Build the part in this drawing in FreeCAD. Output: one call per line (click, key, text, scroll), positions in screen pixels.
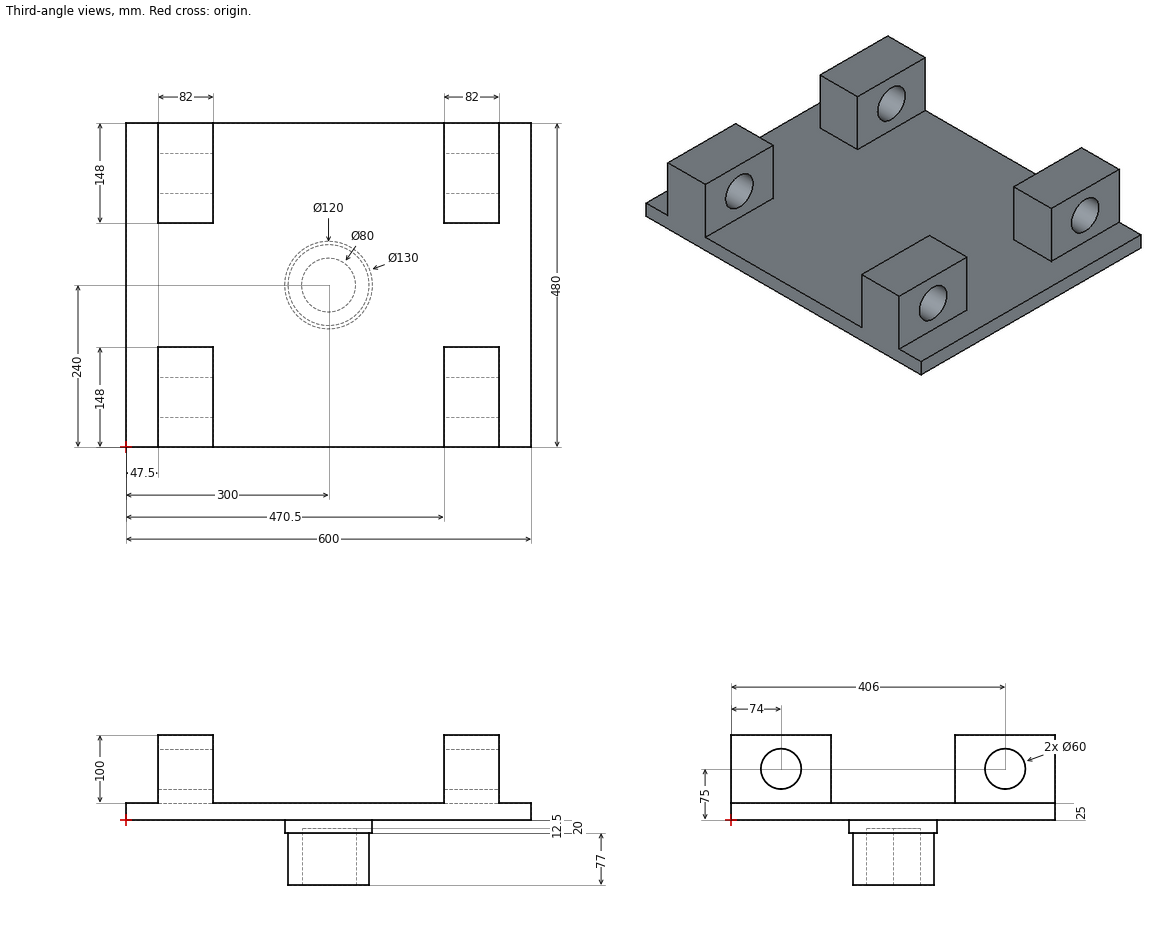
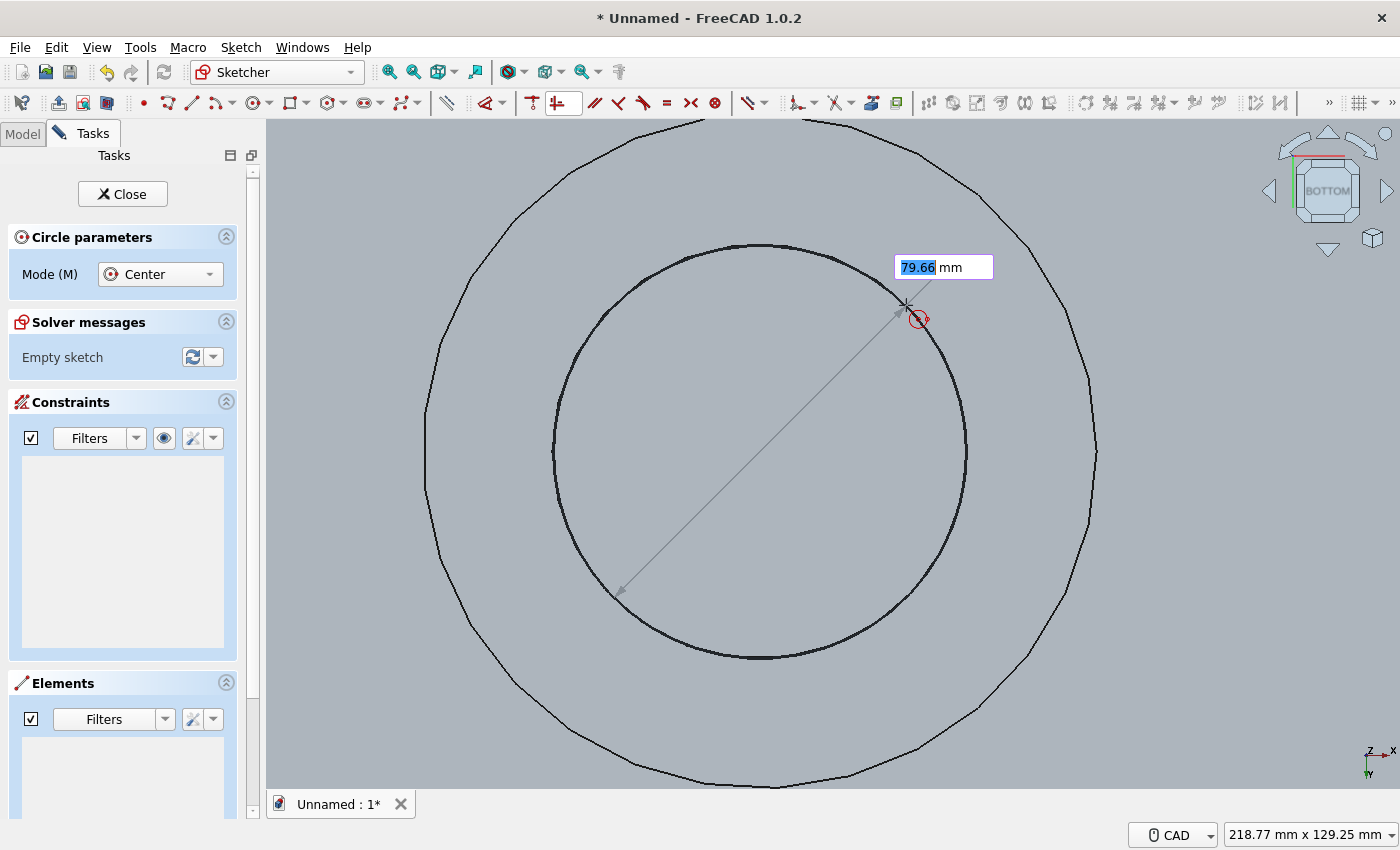
text(80)
key(Return)
key(Escape)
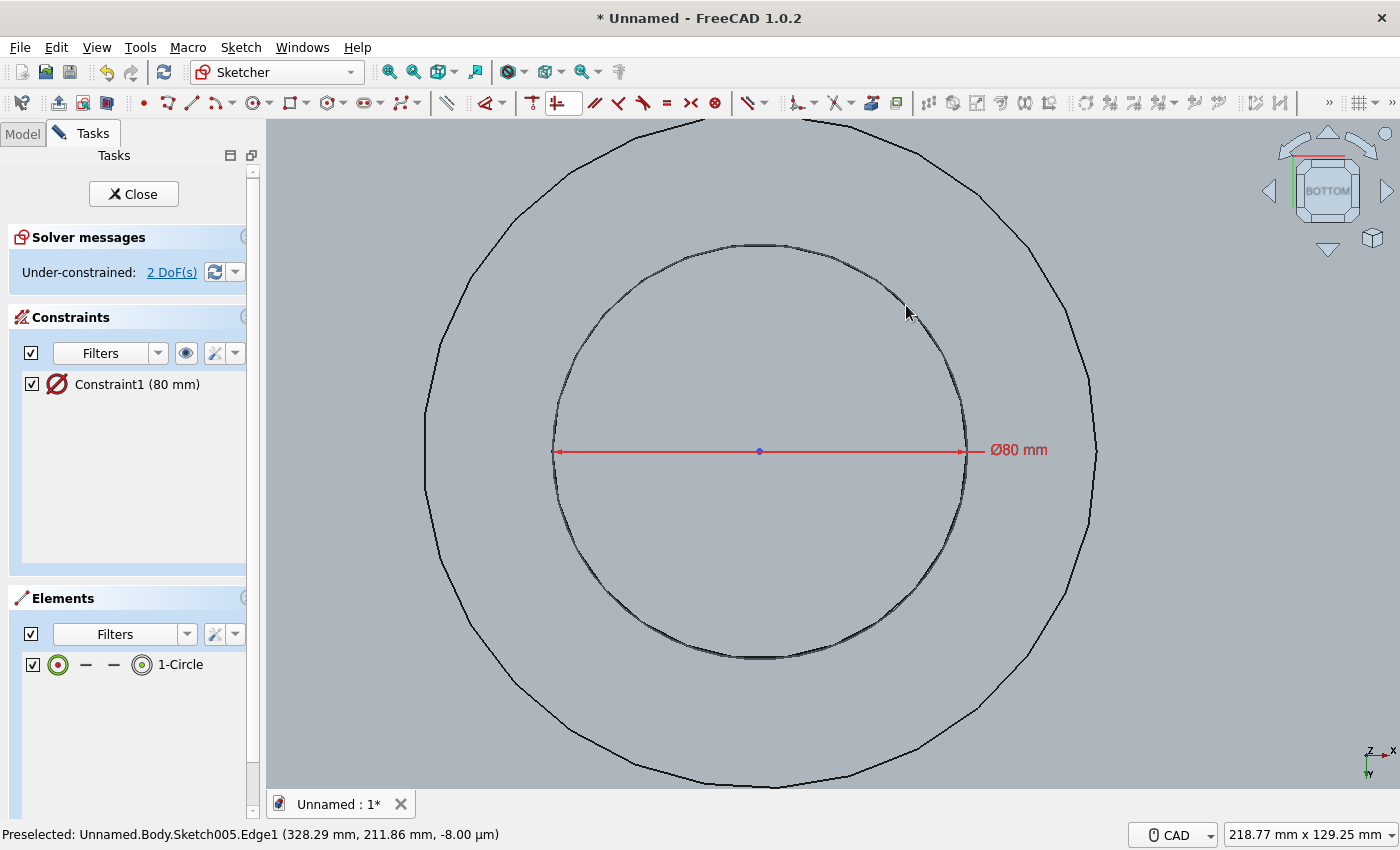
click(486, 104)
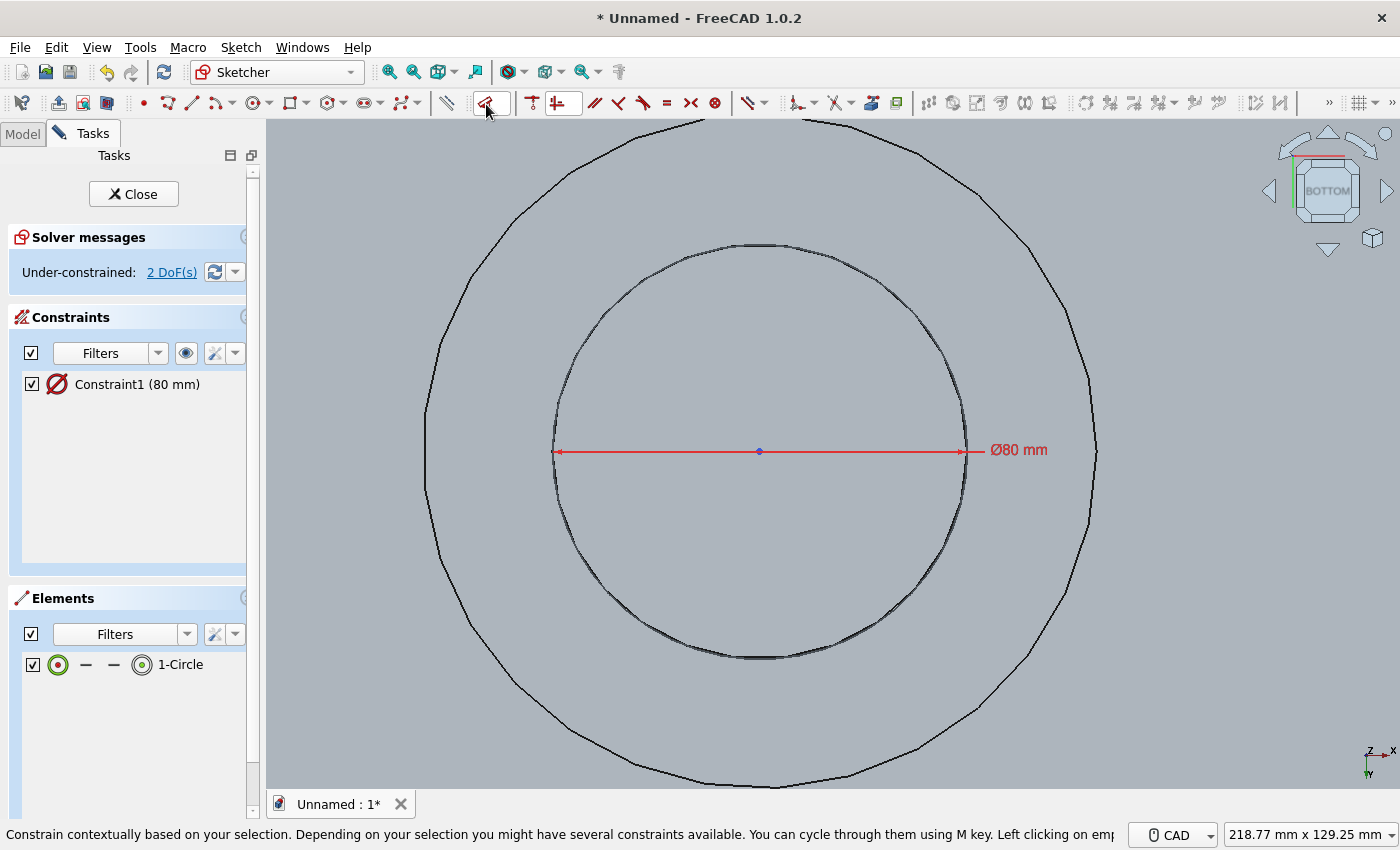
click(760, 452)
click(527, 486)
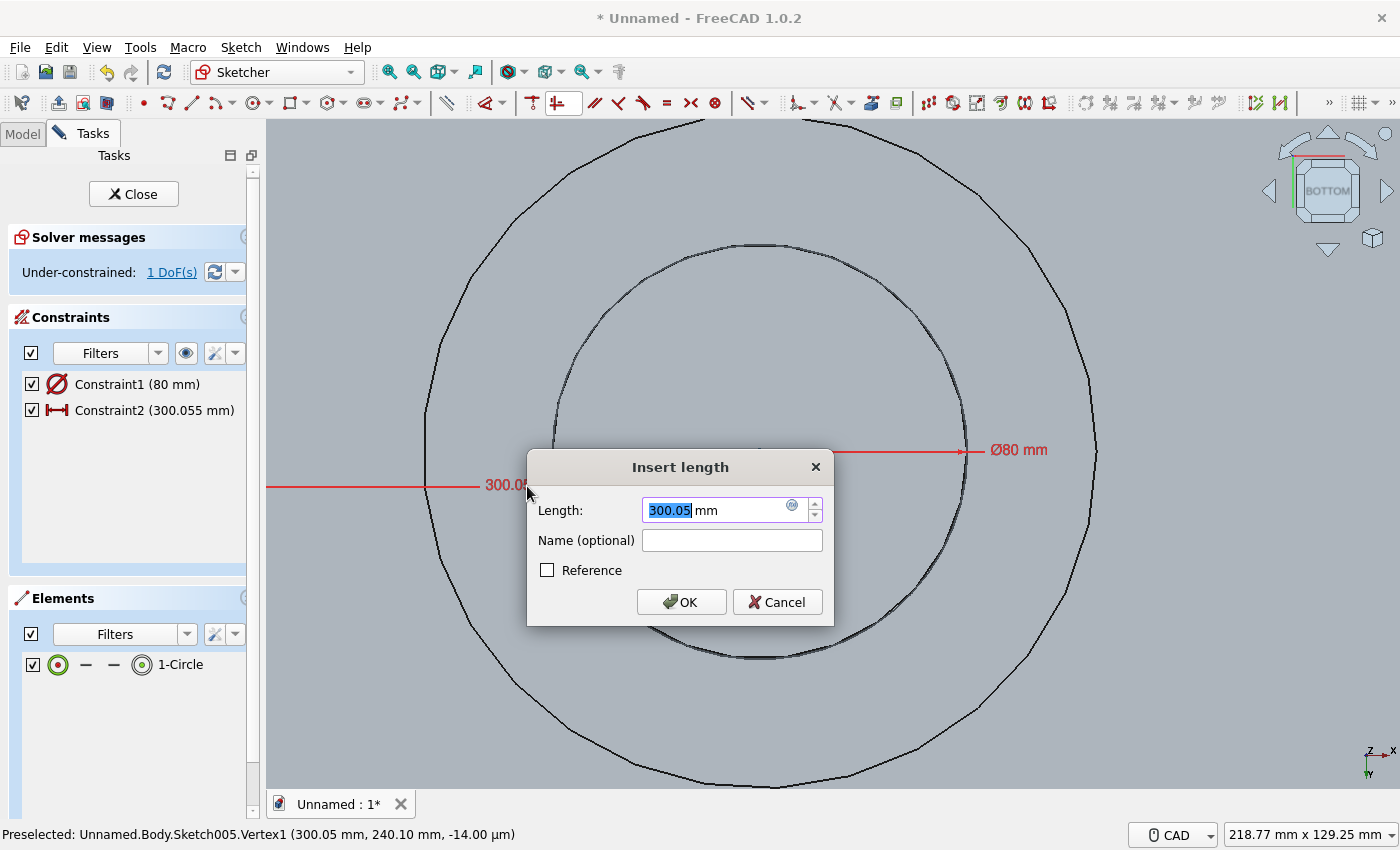
text(300)
key(Return)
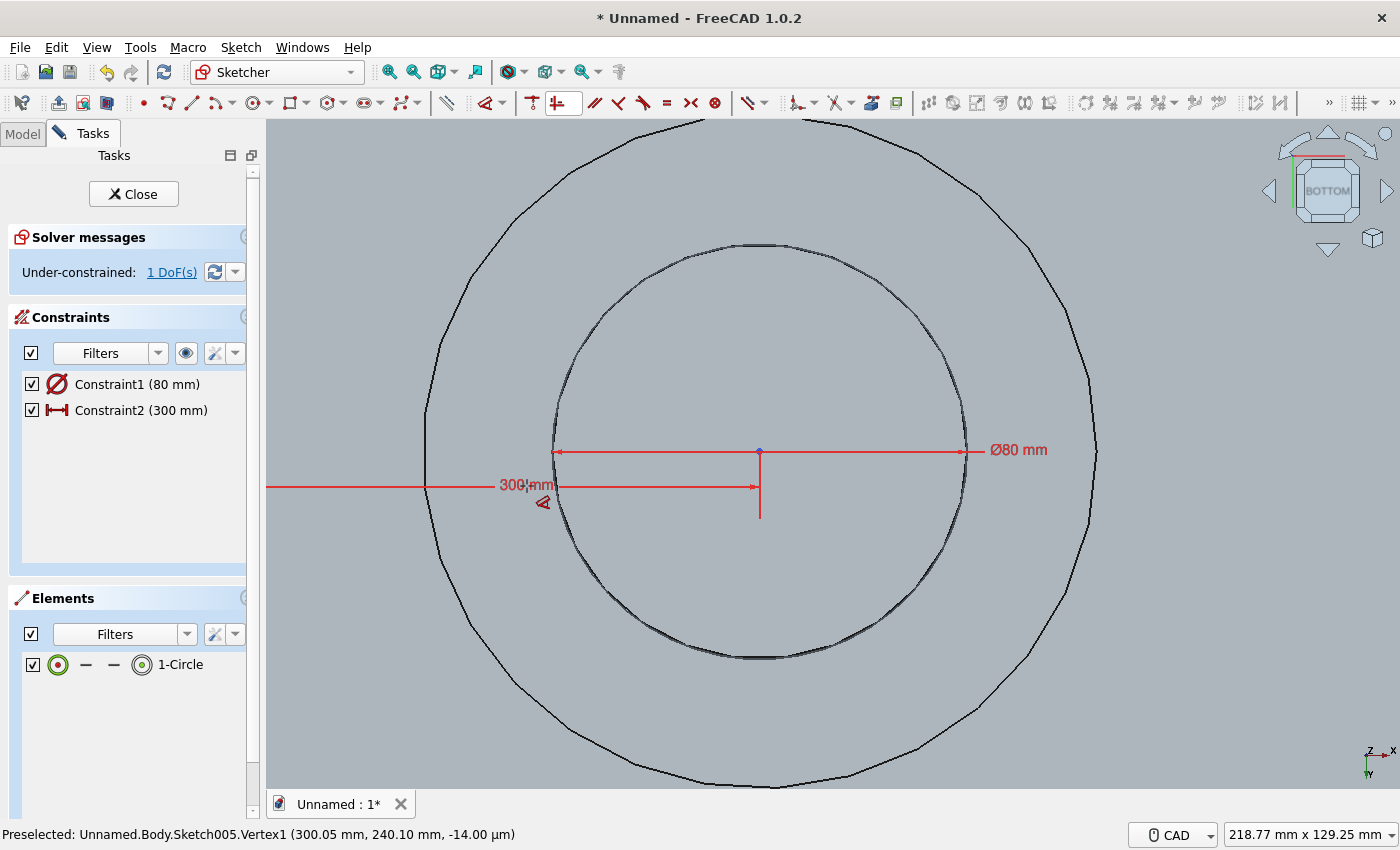
click(760, 452)
click(794, 299)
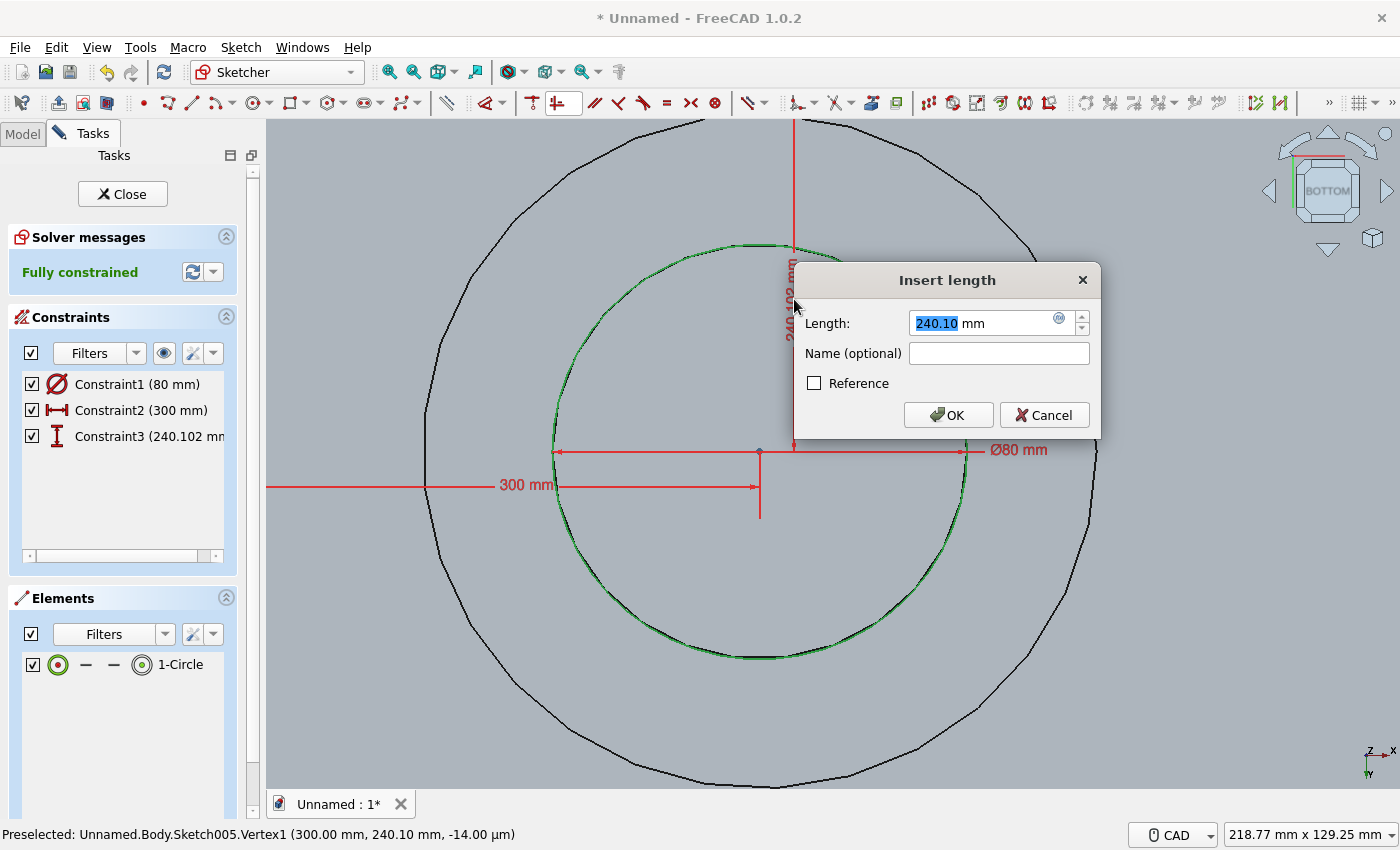
text(240)
key(Return)
key(Escape)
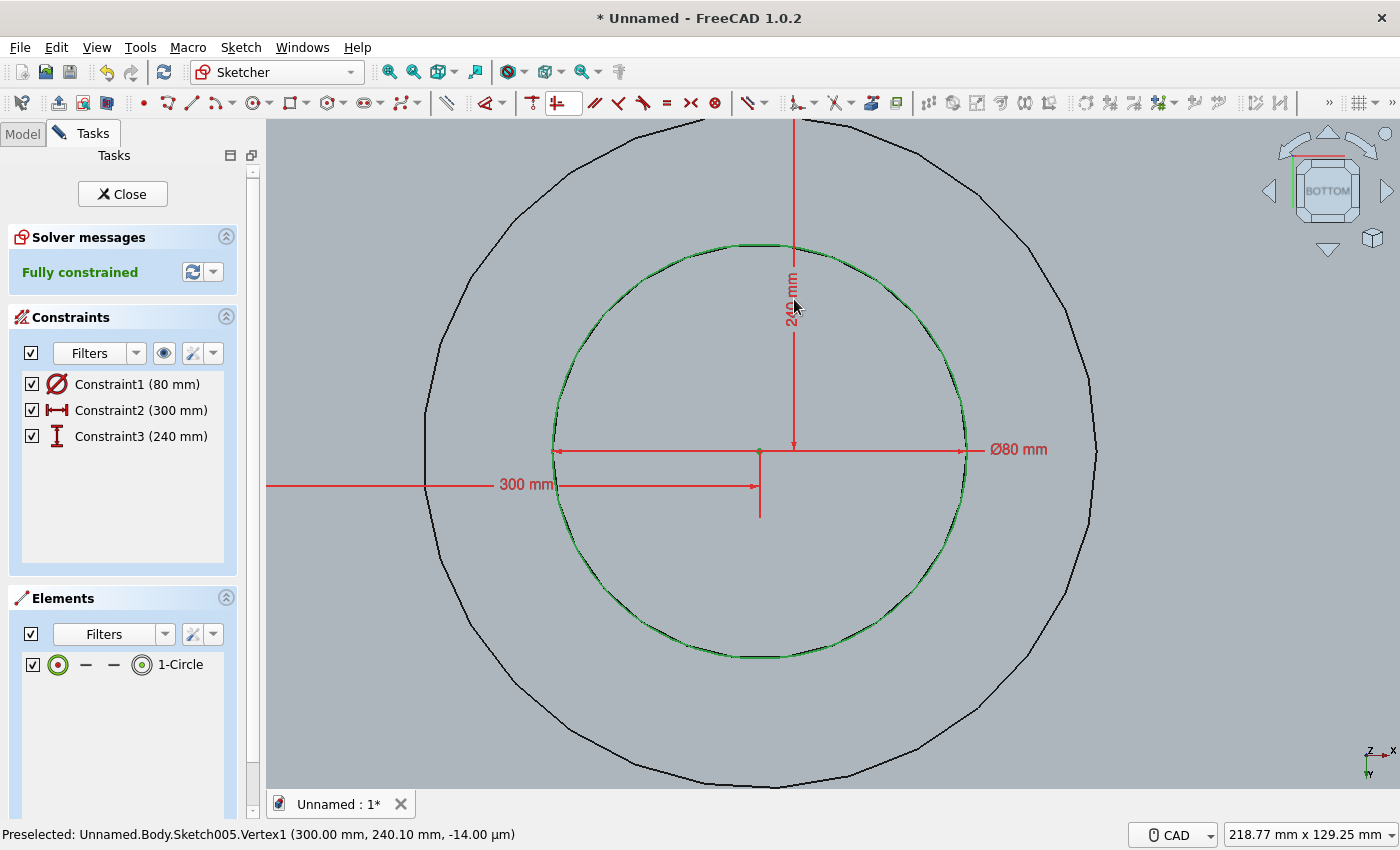
click(123, 194)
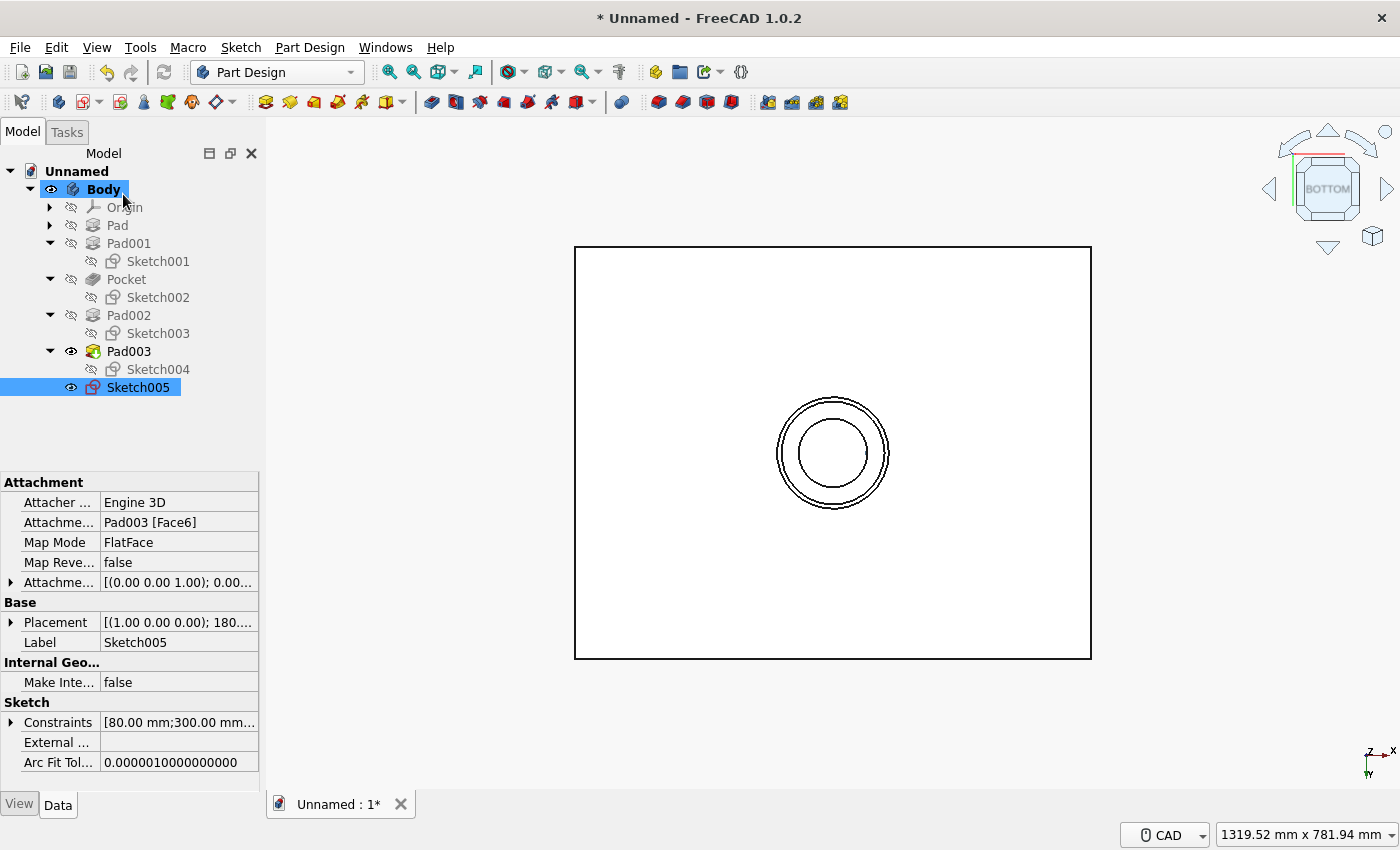
click(266, 102)